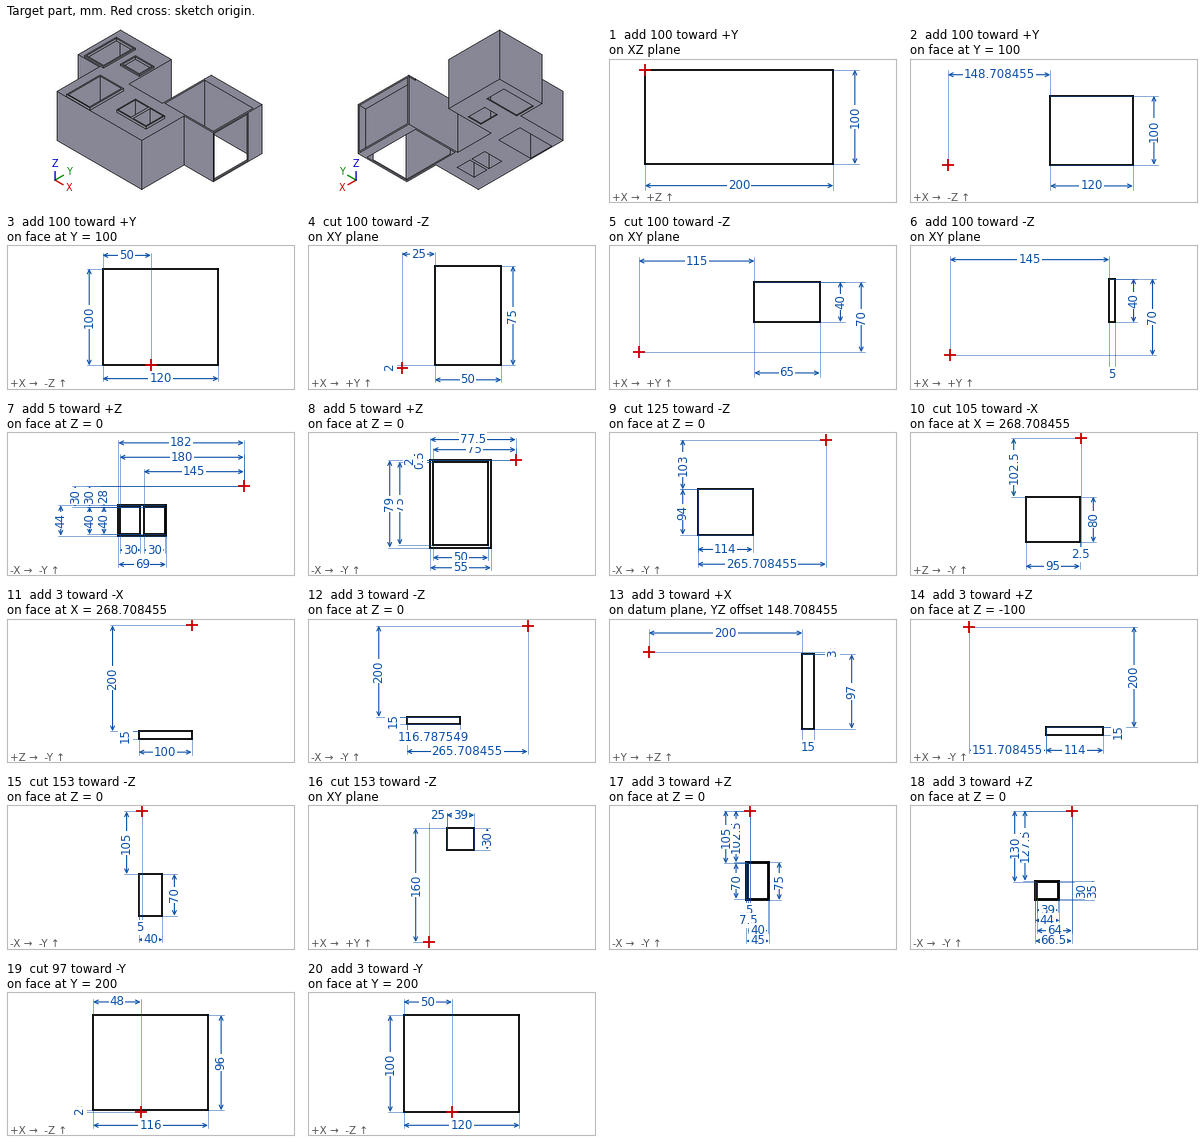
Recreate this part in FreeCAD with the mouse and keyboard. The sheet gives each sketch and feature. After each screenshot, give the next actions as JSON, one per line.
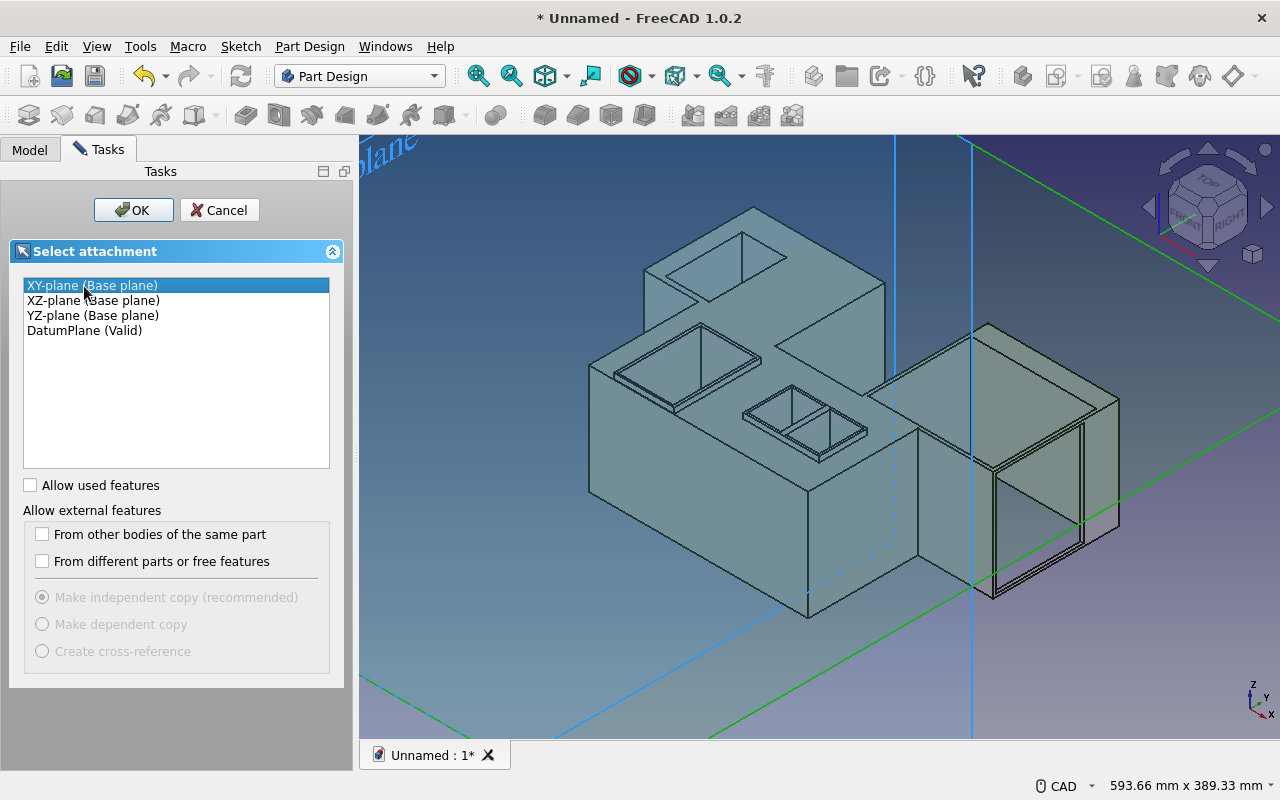
{"action": "left_click", "coordinate": [134, 210]}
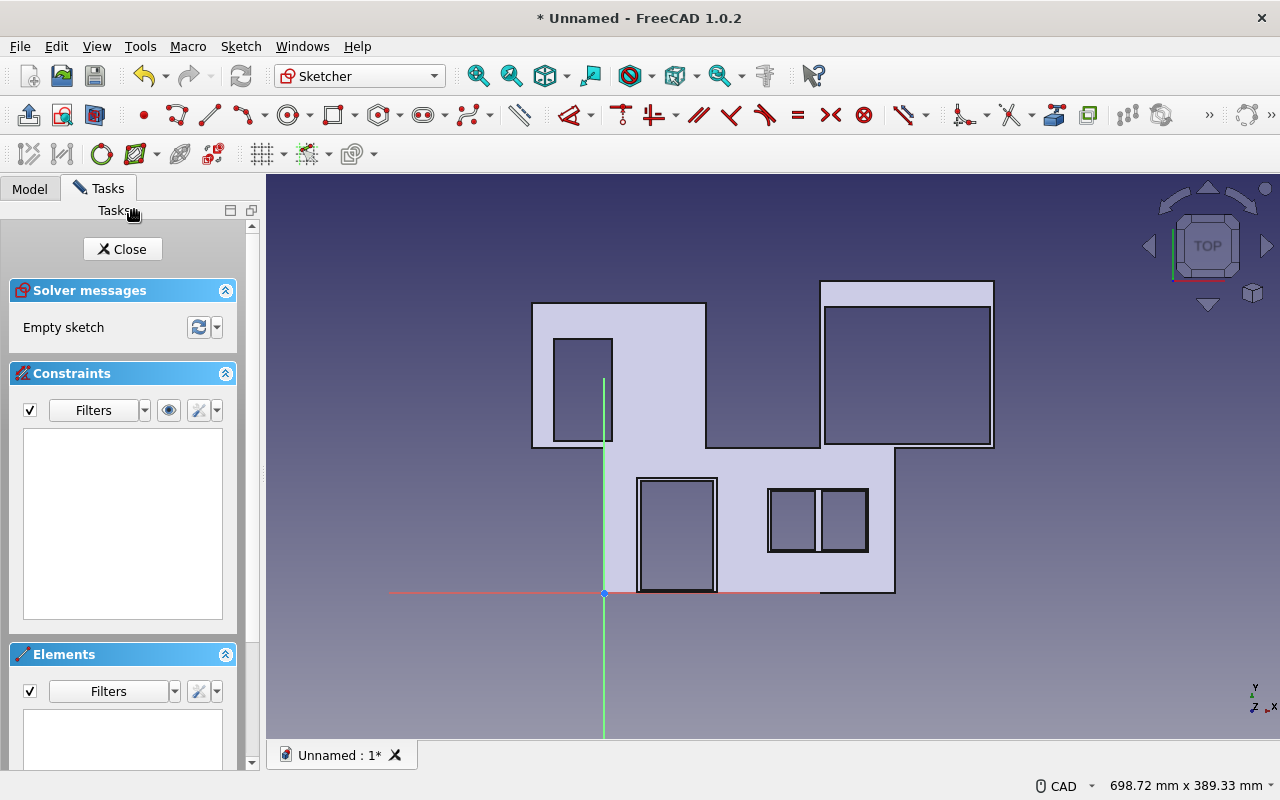
{"action": "left_click", "coordinate": [95, 116]}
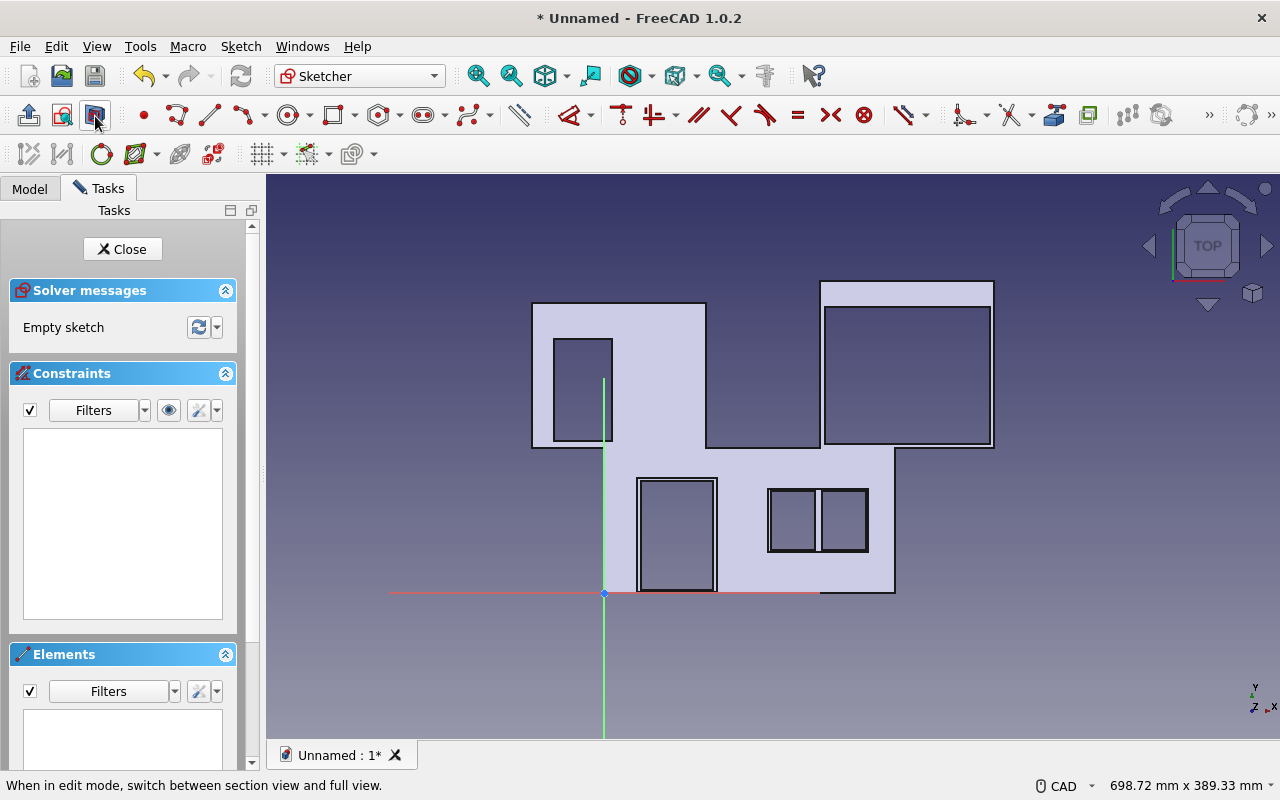
{"action": "scroll", "coordinate": [665, 373], "scroll_direction": "up", "scroll_amount": 11}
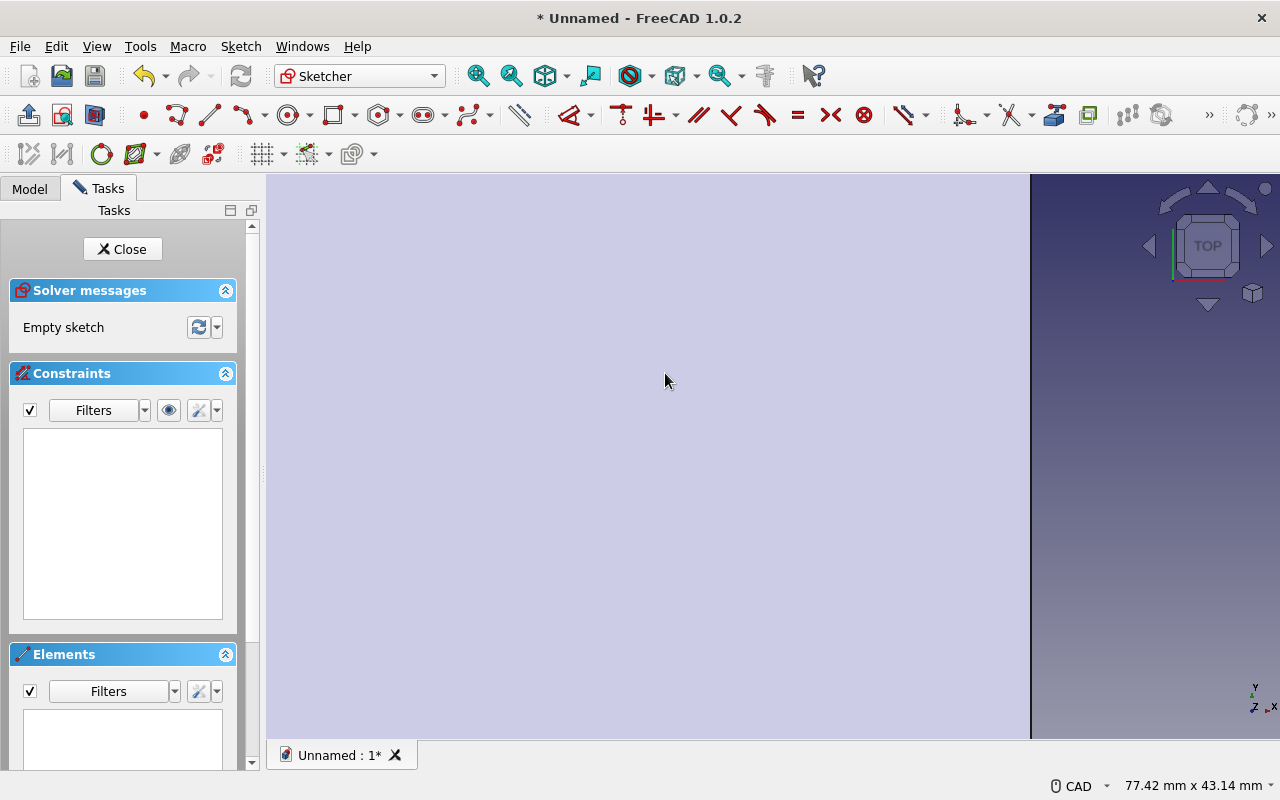
{"action": "left_click", "coordinate": [332, 116]}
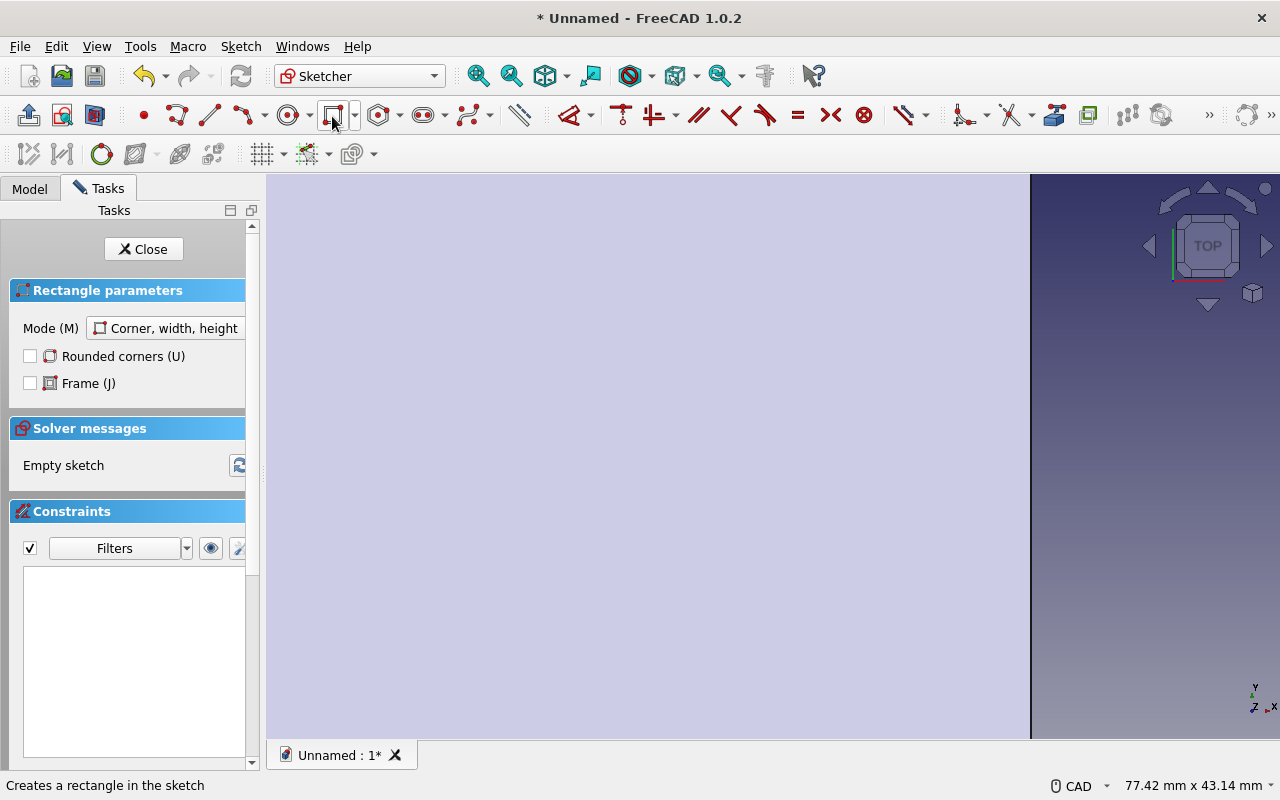
{"action": "left_click", "coordinate": [442, 261]}
{"action": "mouse_move", "coordinate": [953, 654]}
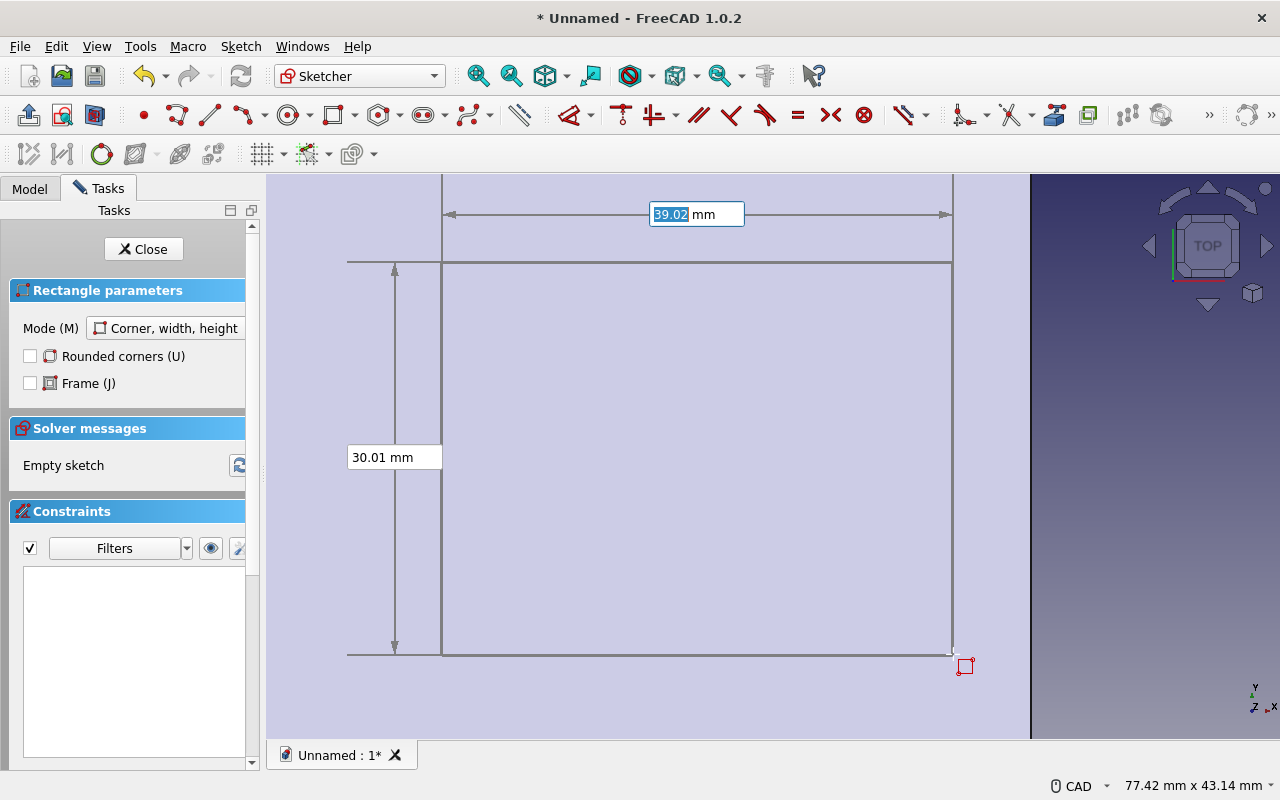
{"action": "type", "text": "39"}
{"action": "key", "text": "Tab"}
{"action": "type", "text": "30"}
{"action": "key", "text": "Return"}
{"action": "key", "text": "Escape"}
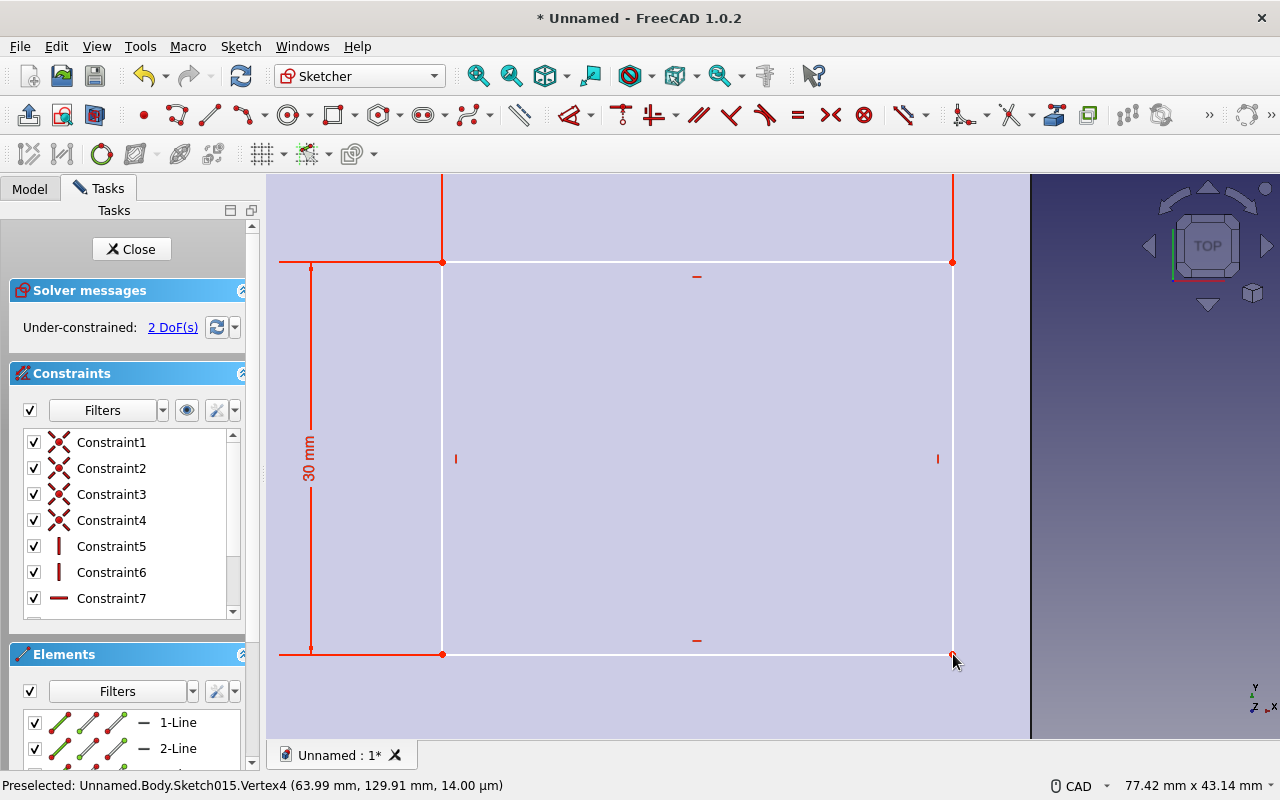
{"action": "left_click", "coordinate": [568, 116]}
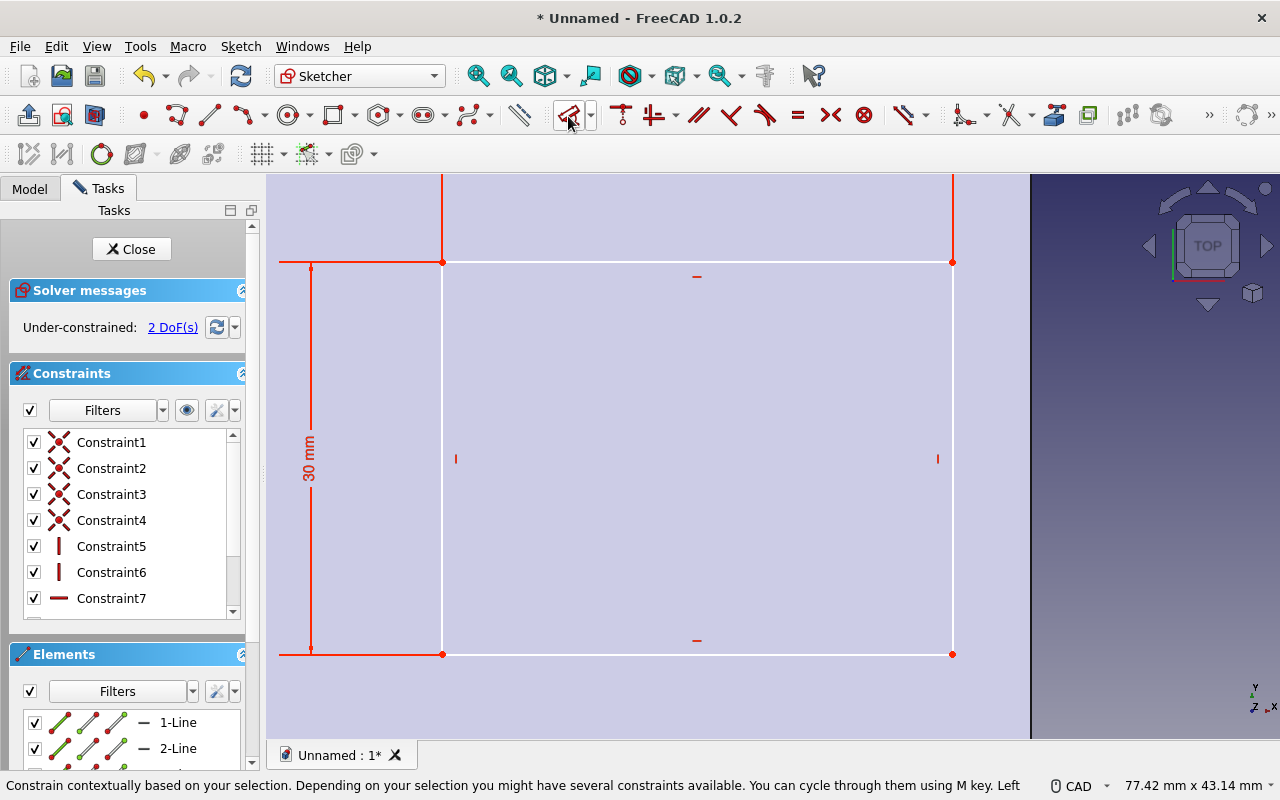
{"action": "left_click", "coordinate": [442, 262]}
{"action": "left_click", "coordinate": [368, 228]}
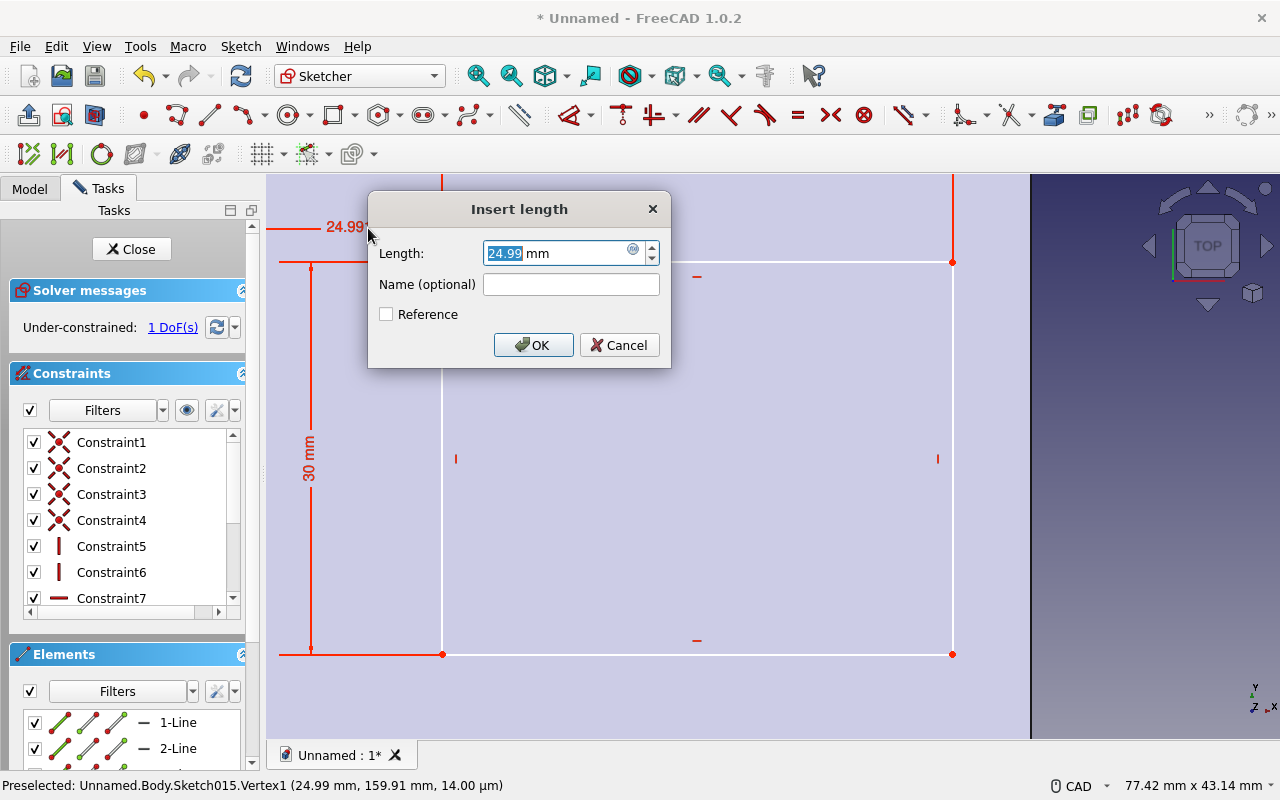
{"action": "type", "text": "25"}
{"action": "key", "text": "Return"}